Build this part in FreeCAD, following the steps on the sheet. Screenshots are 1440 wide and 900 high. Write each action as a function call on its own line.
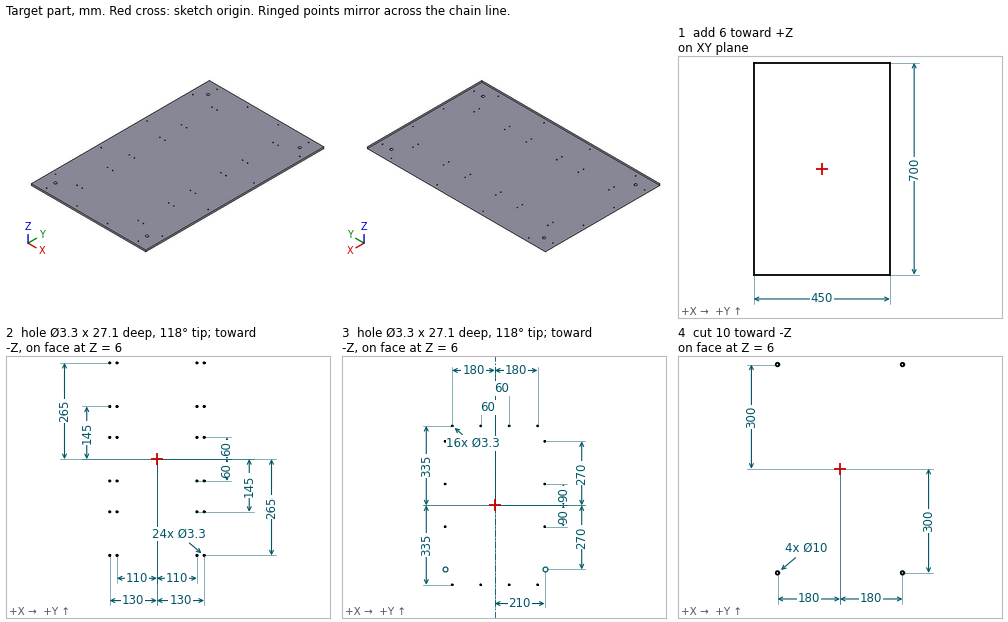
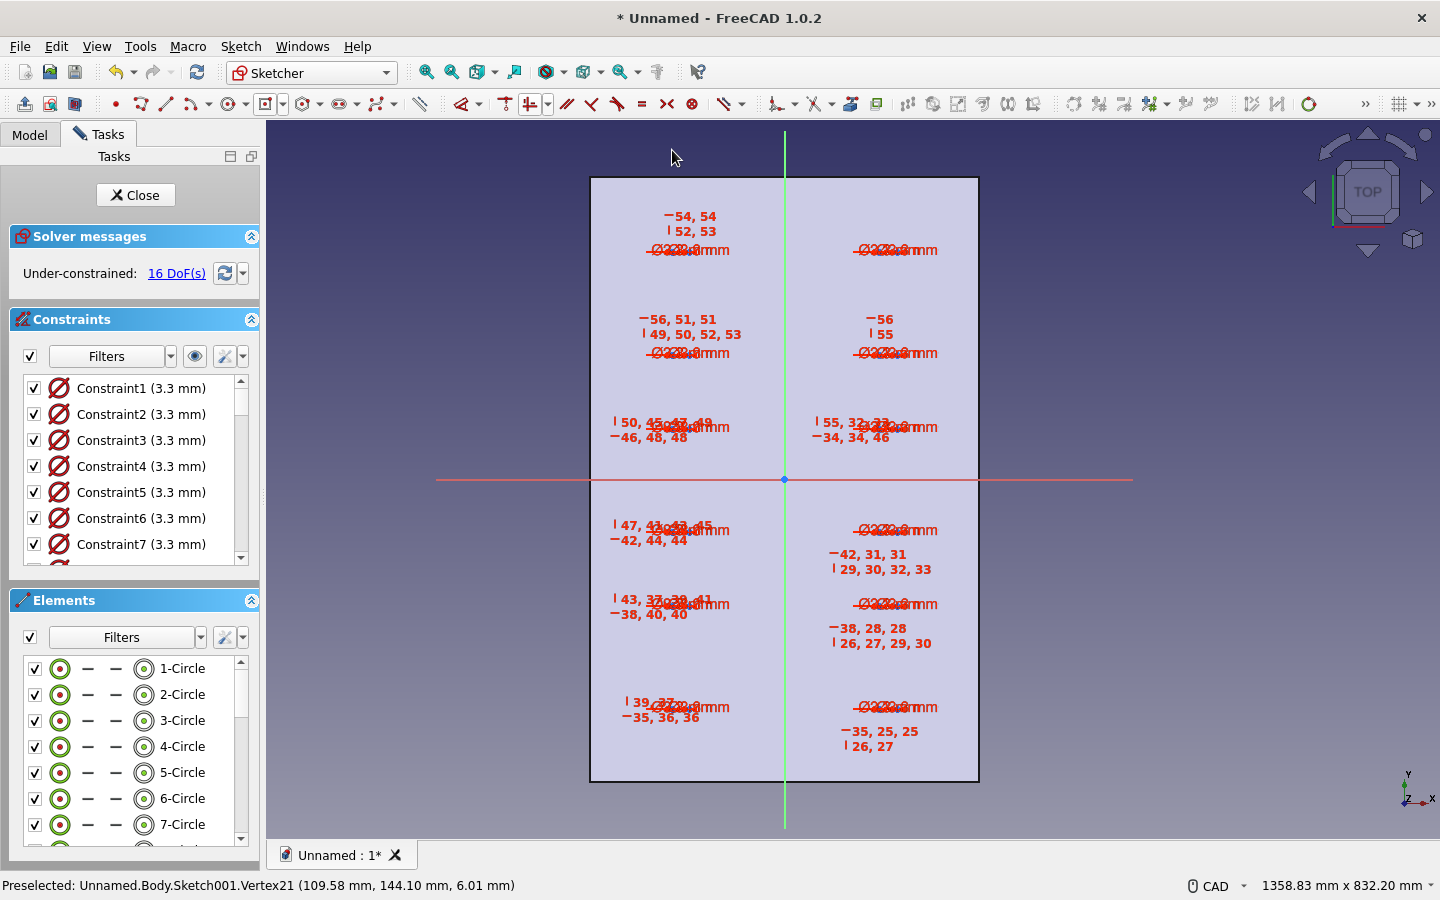
click(897, 429)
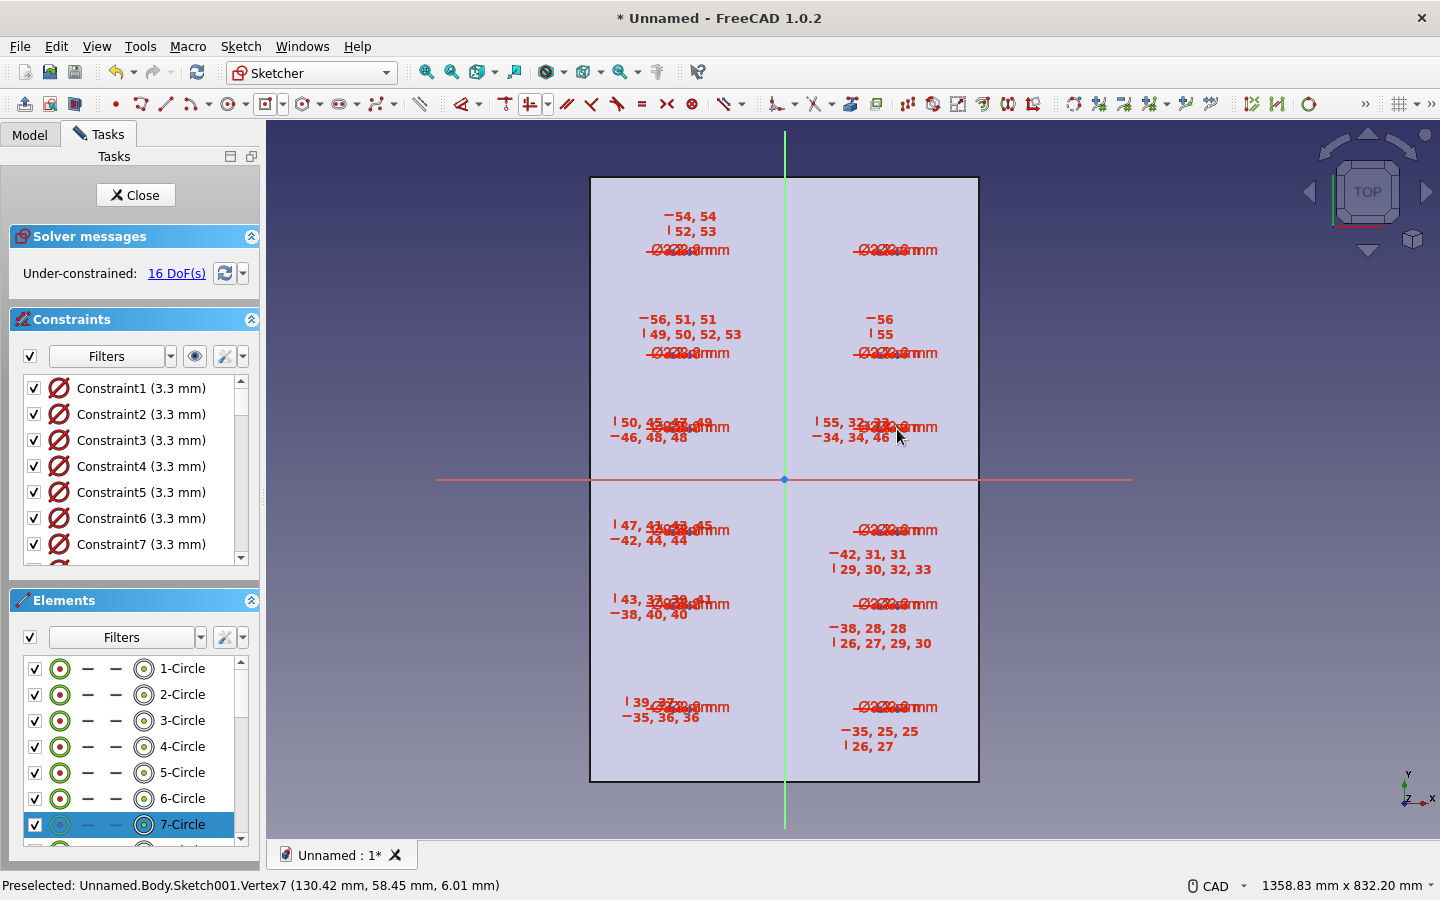
click(897, 355)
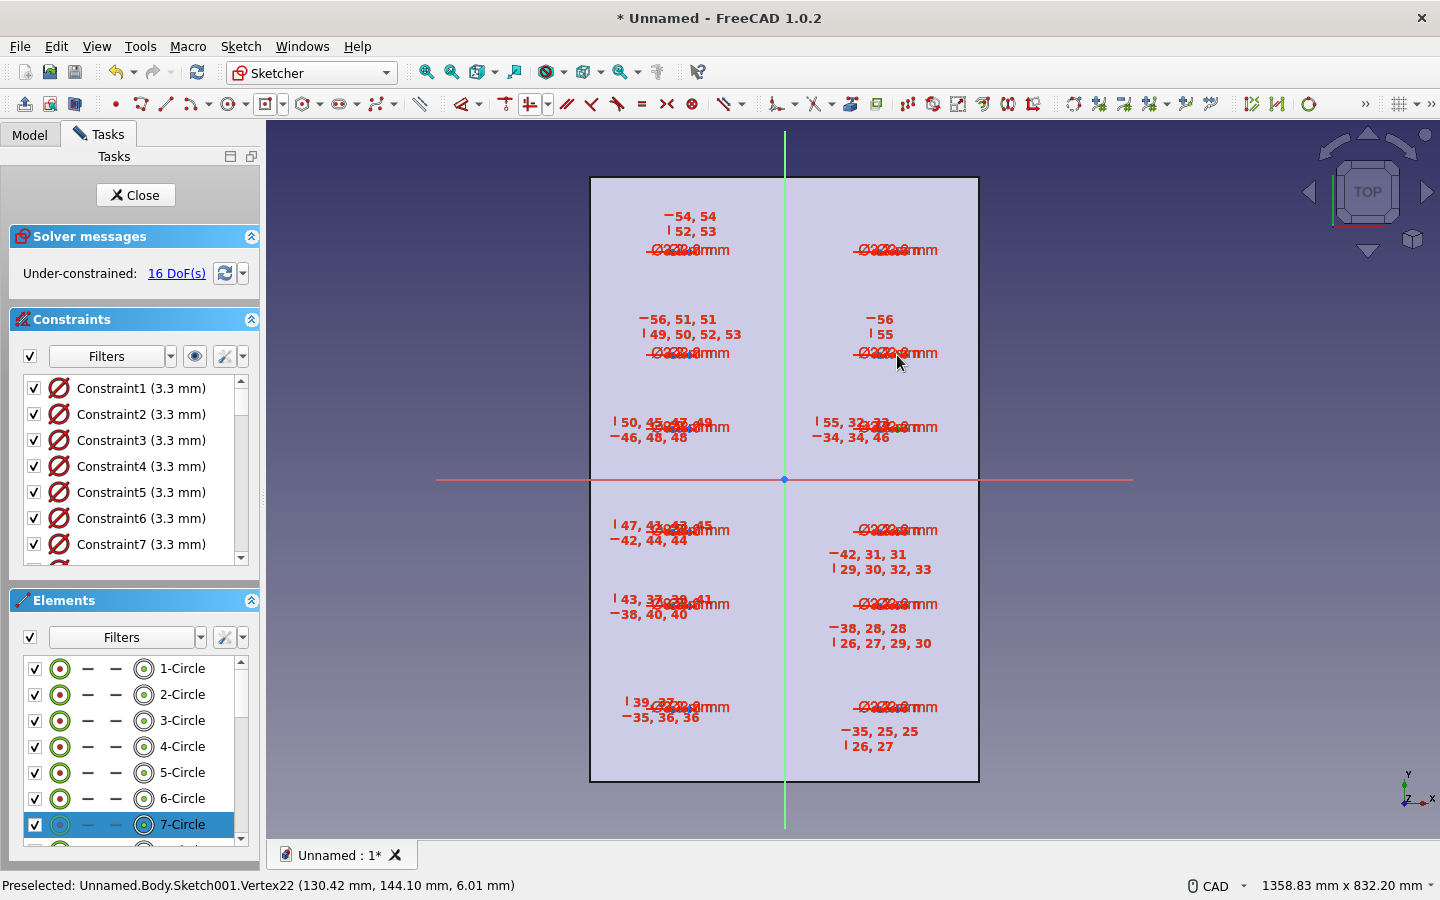
key(v)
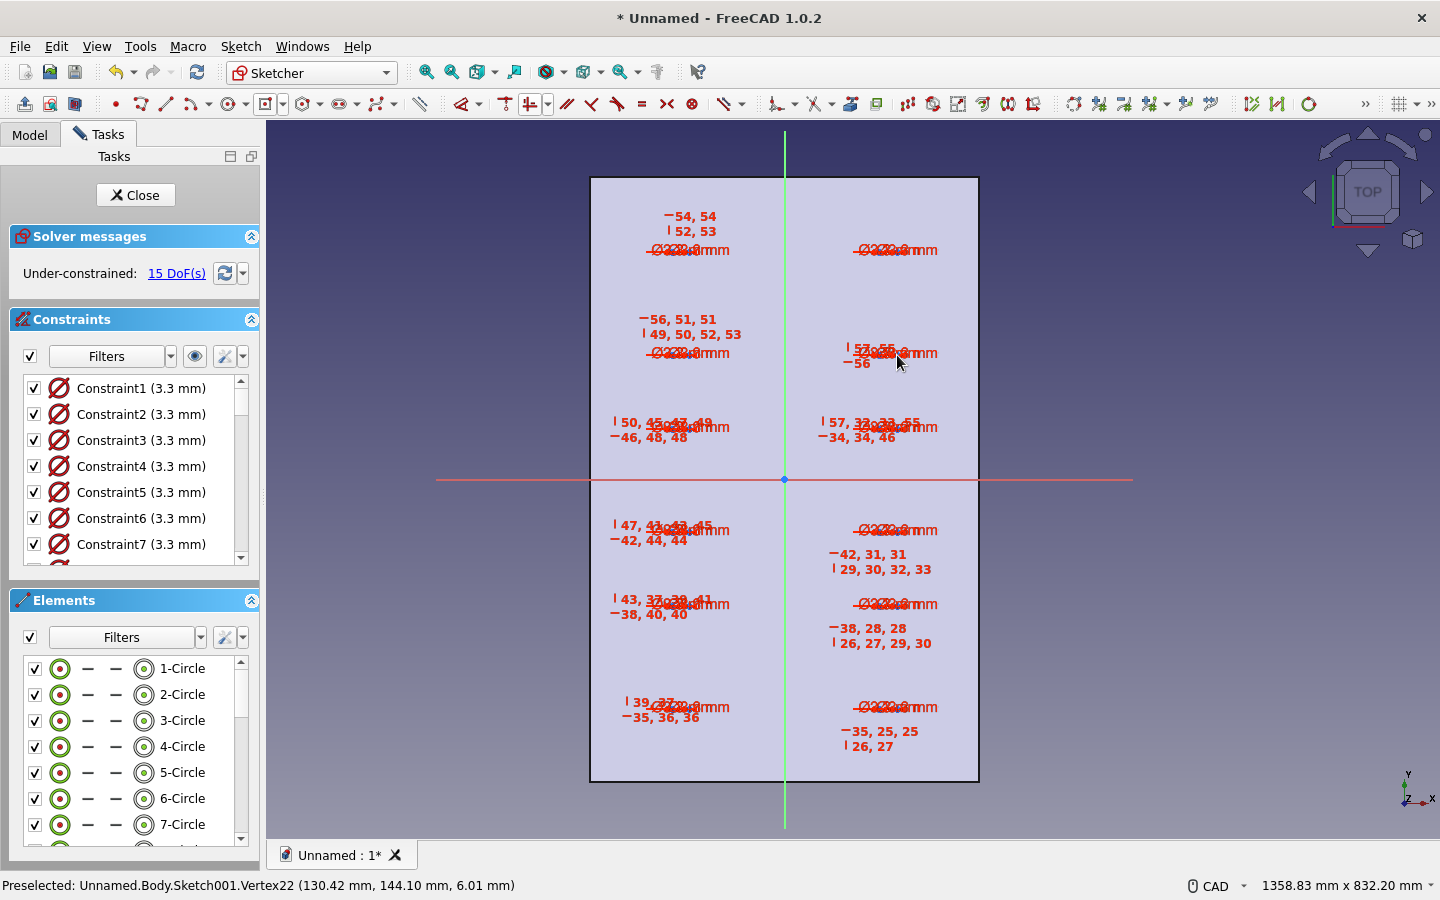
scroll(879, 355, up, 4)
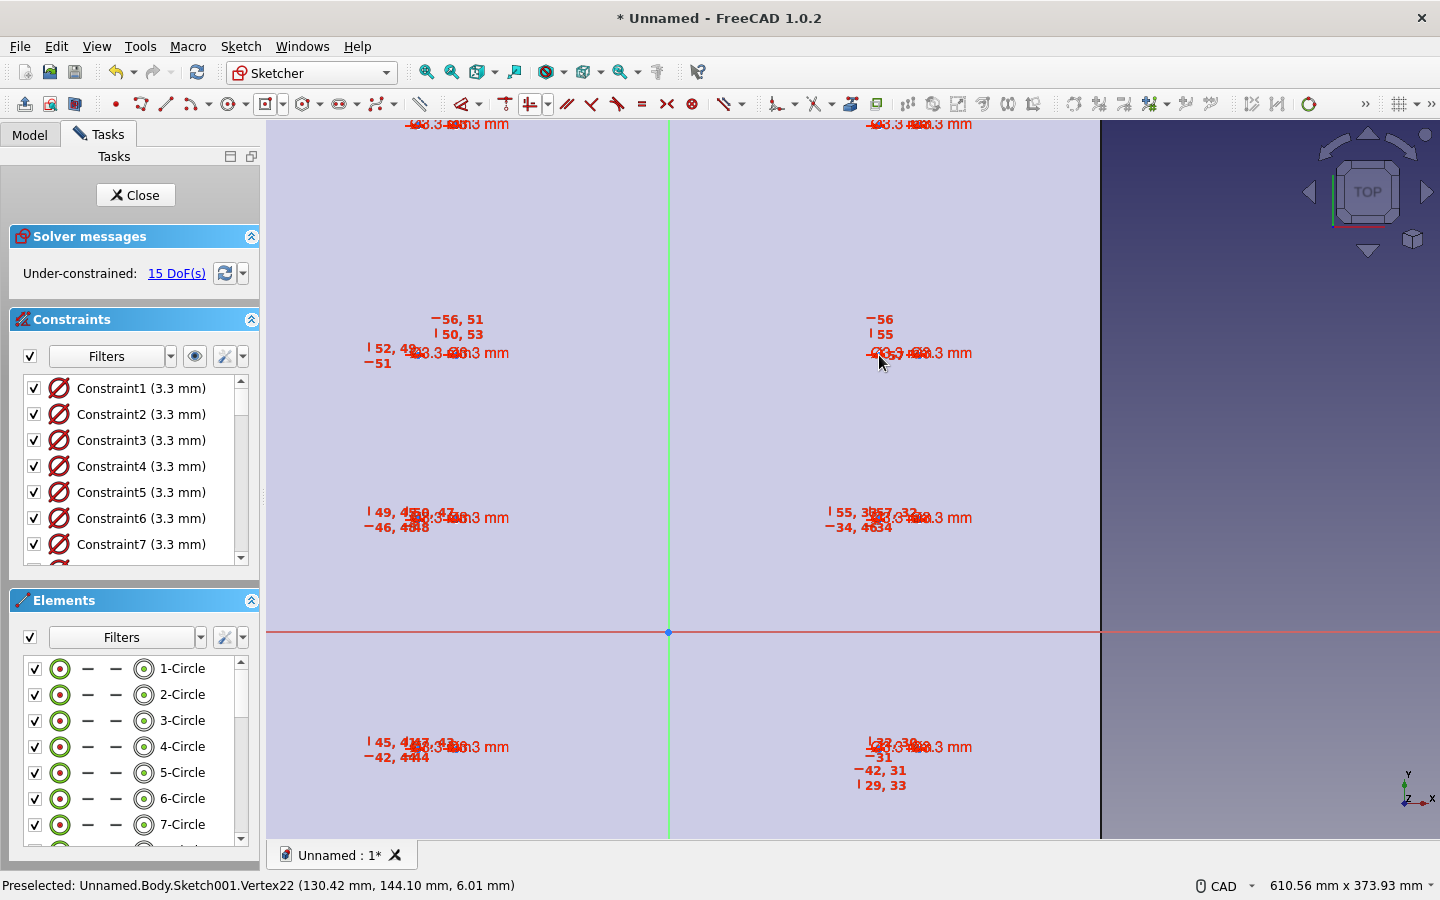
scroll(879, 355, up, 4)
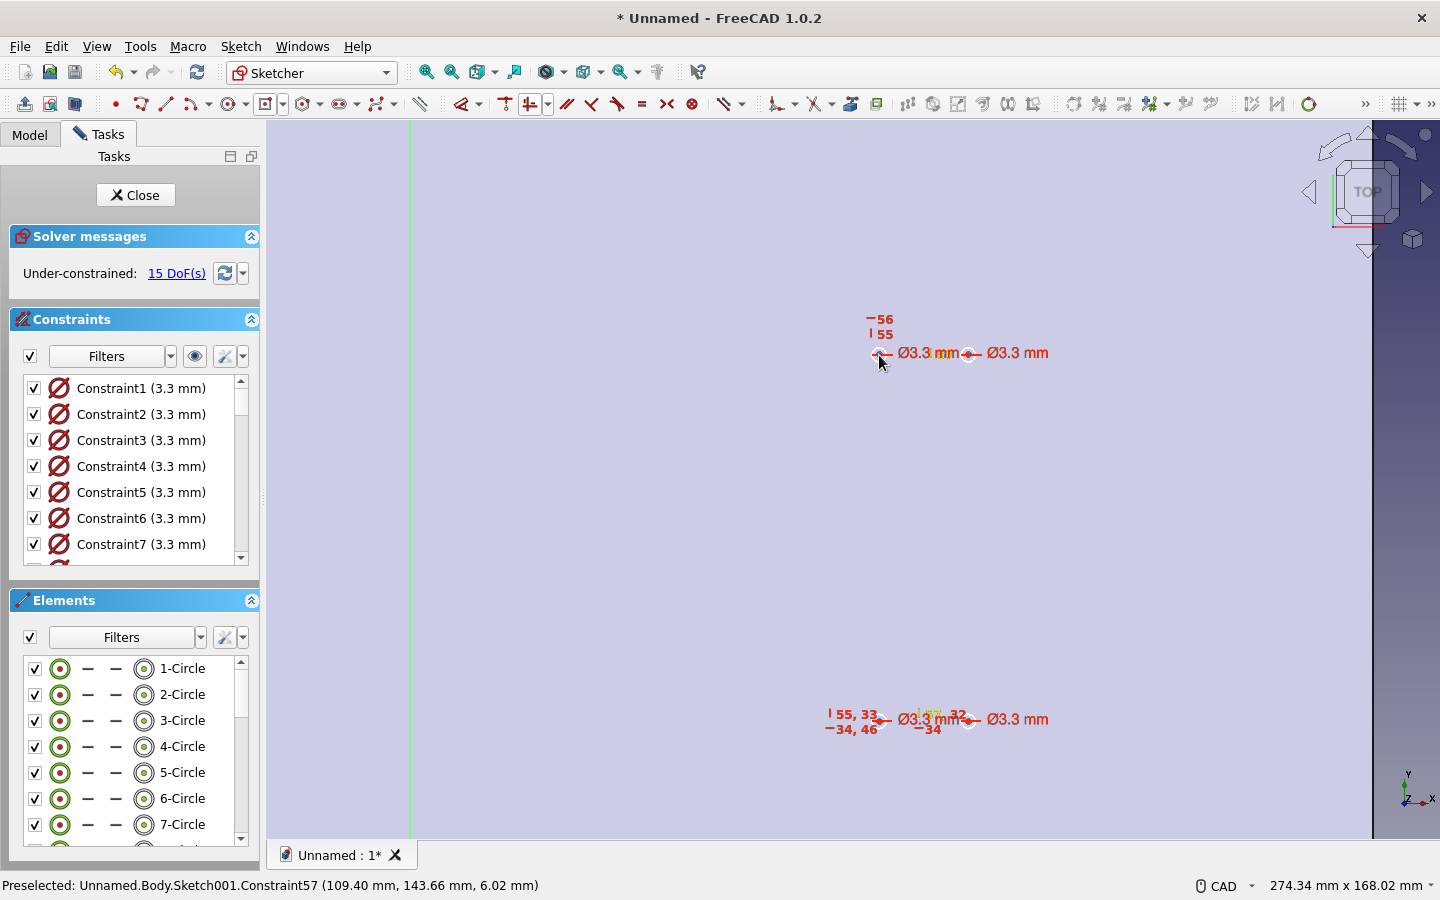
click(879, 355)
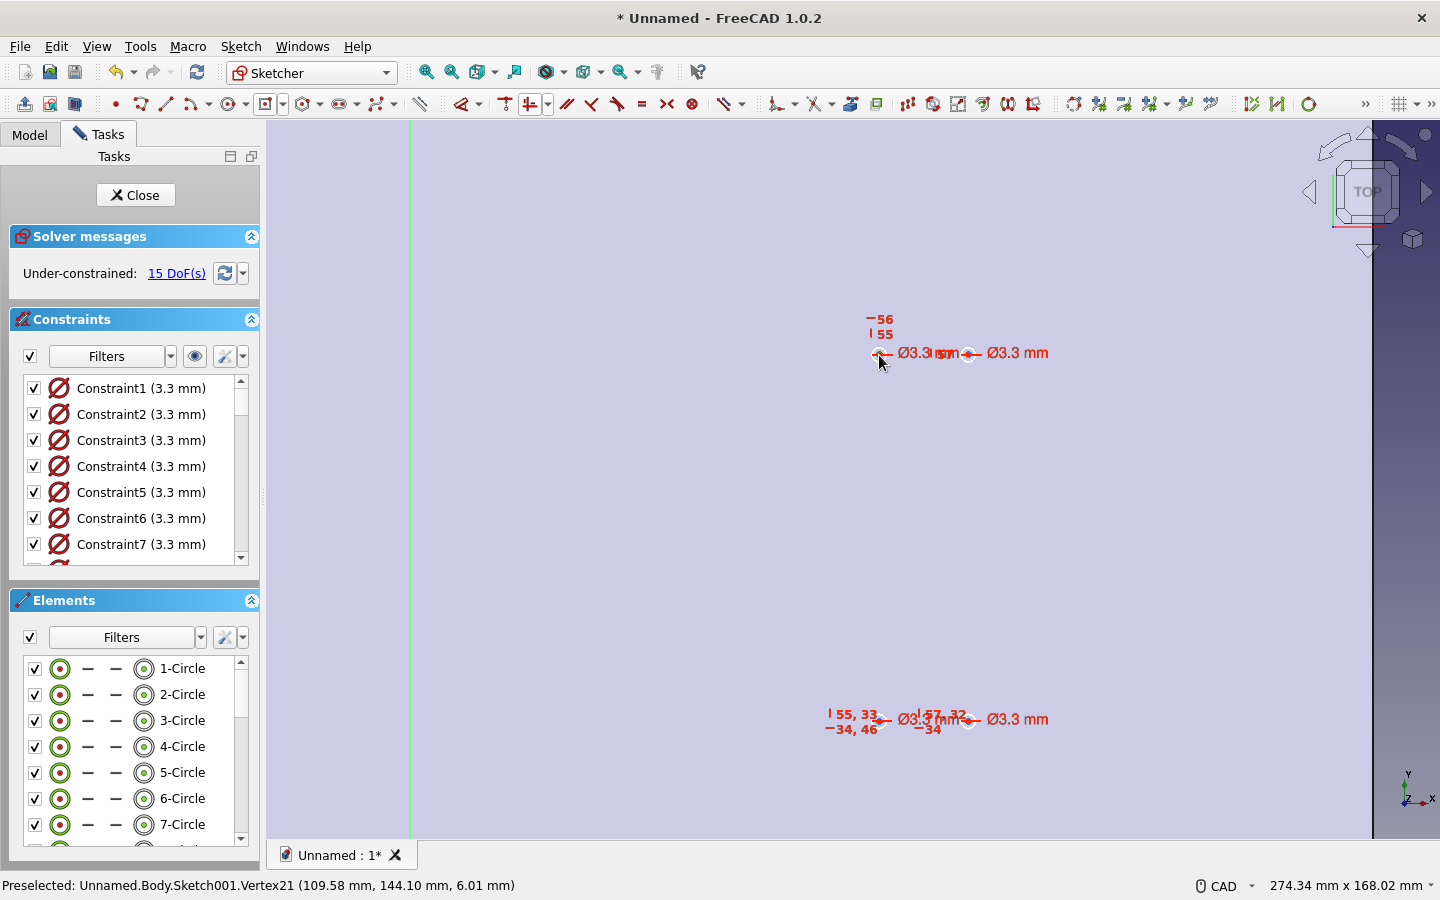
scroll(879, 355, down, 8)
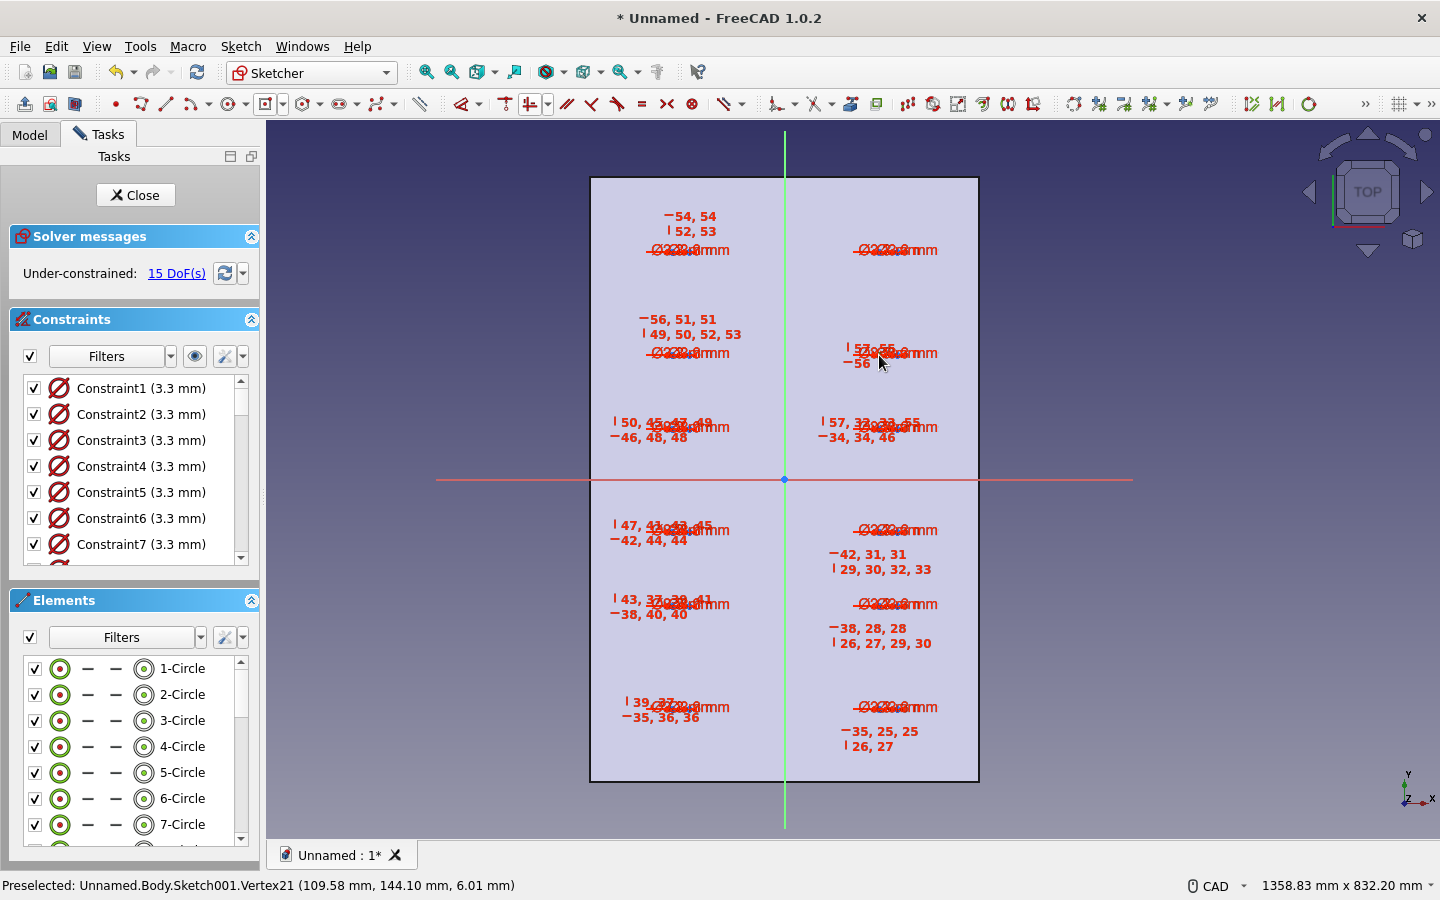
click(897, 355)